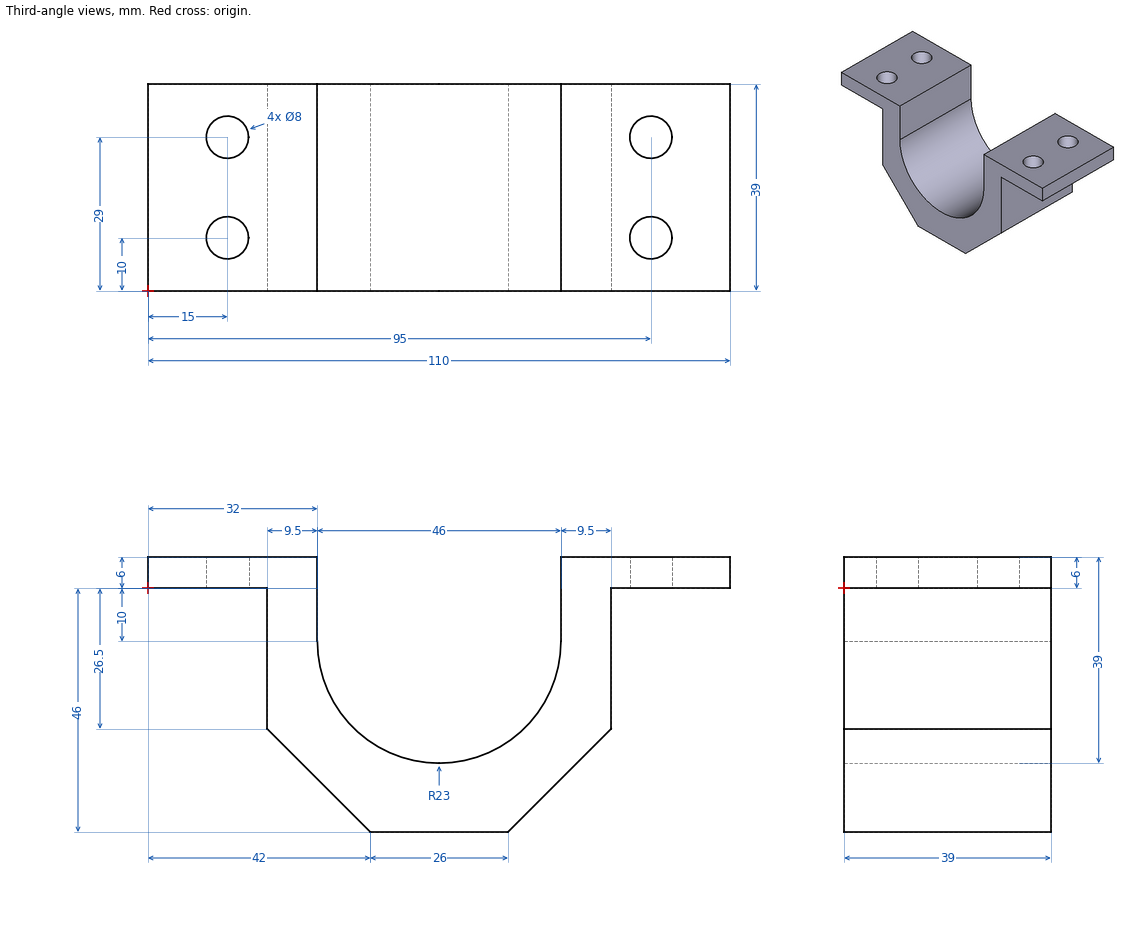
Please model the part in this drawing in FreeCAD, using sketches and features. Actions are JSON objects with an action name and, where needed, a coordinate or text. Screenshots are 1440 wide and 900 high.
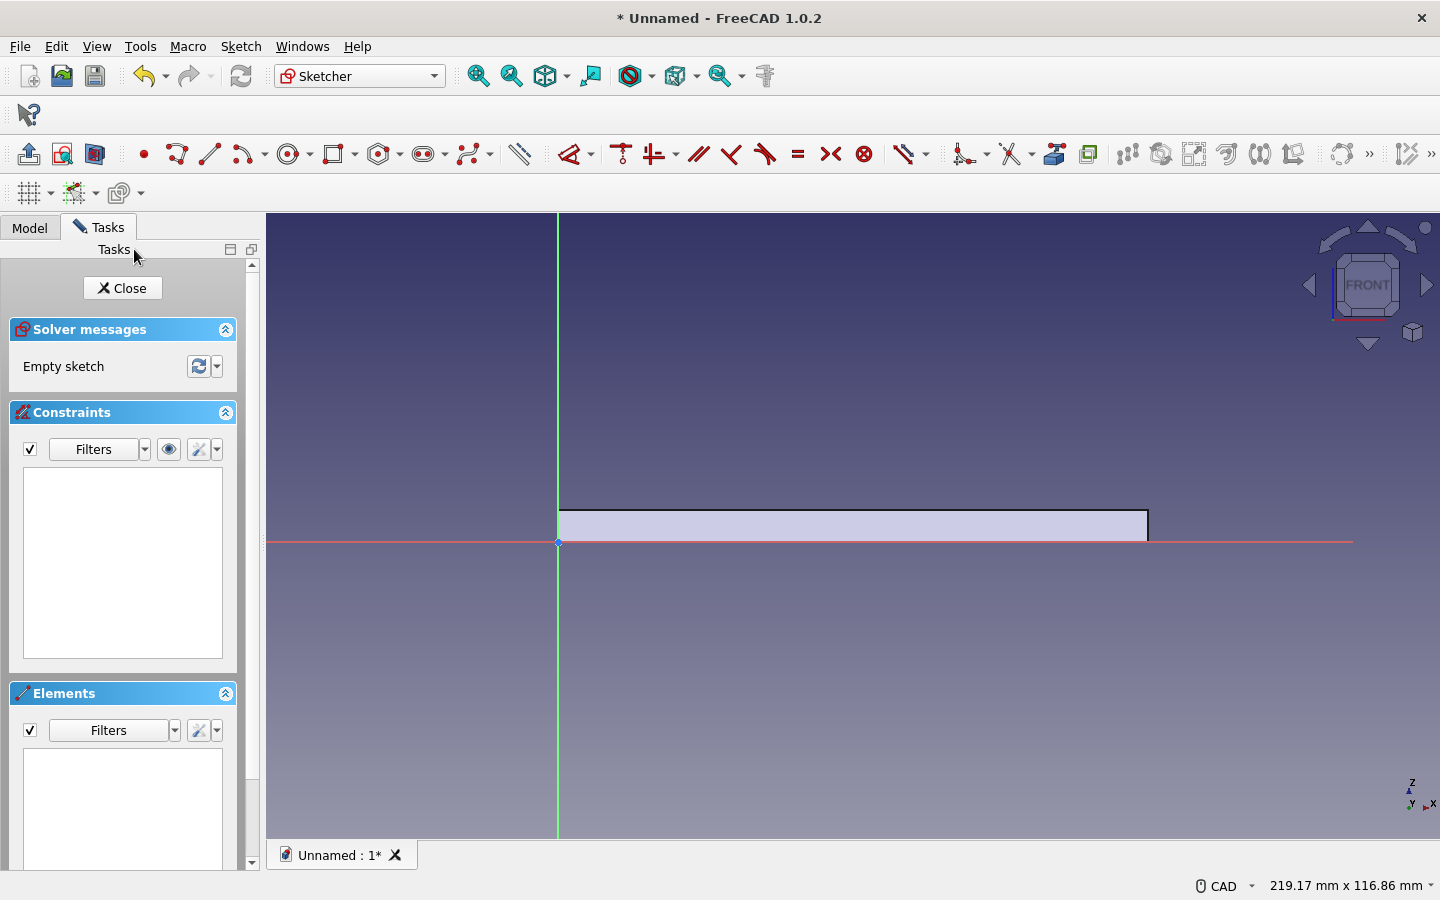
{"action": "scroll", "coordinate": [809, 811], "scroll_direction": "up", "scroll_amount": 2}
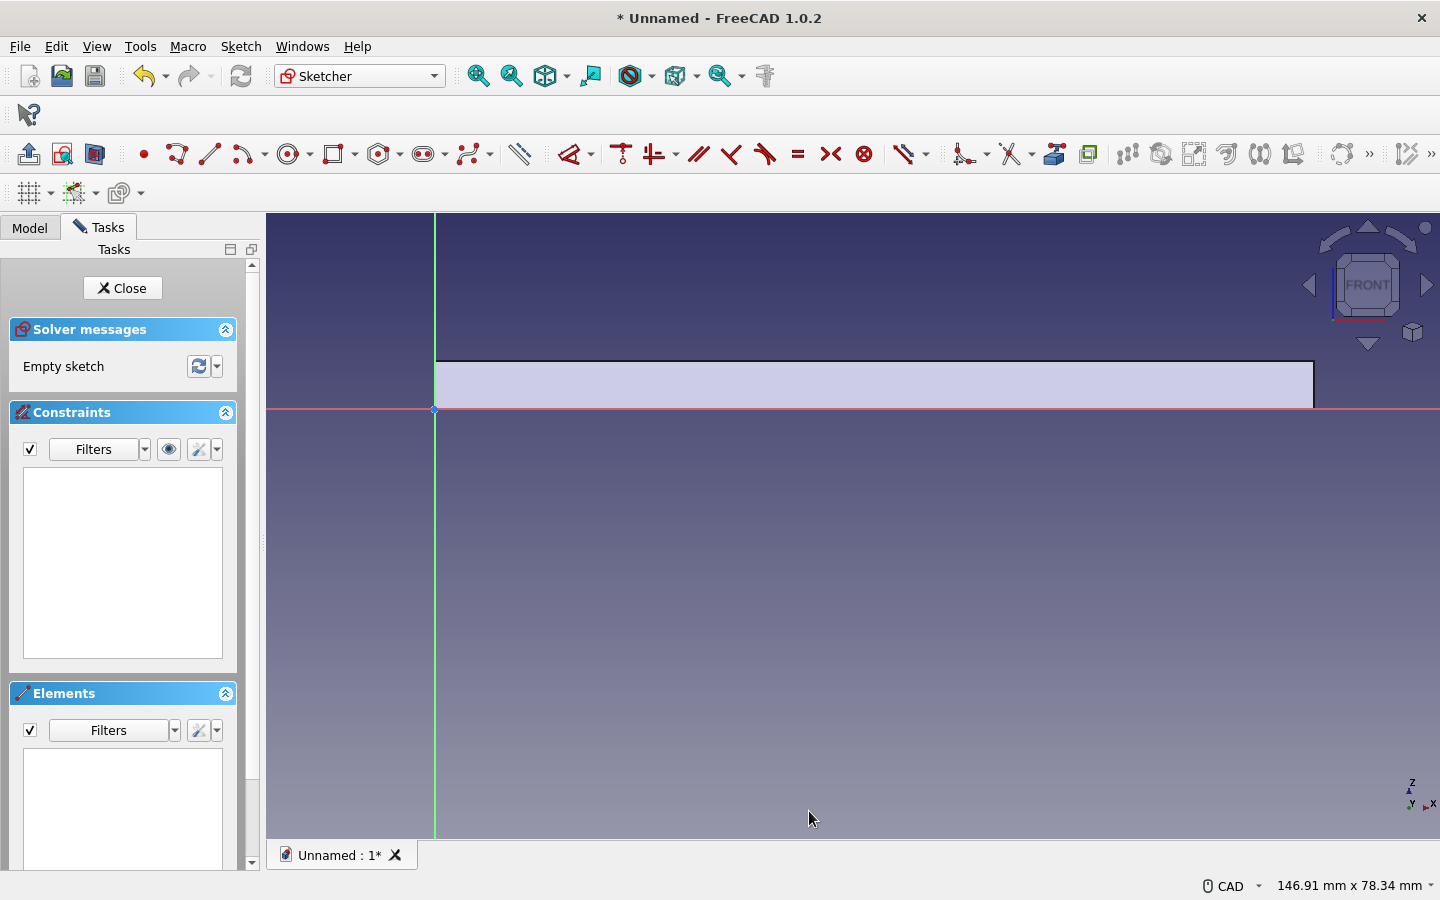
{"action": "left_click", "coordinate": [177, 154]}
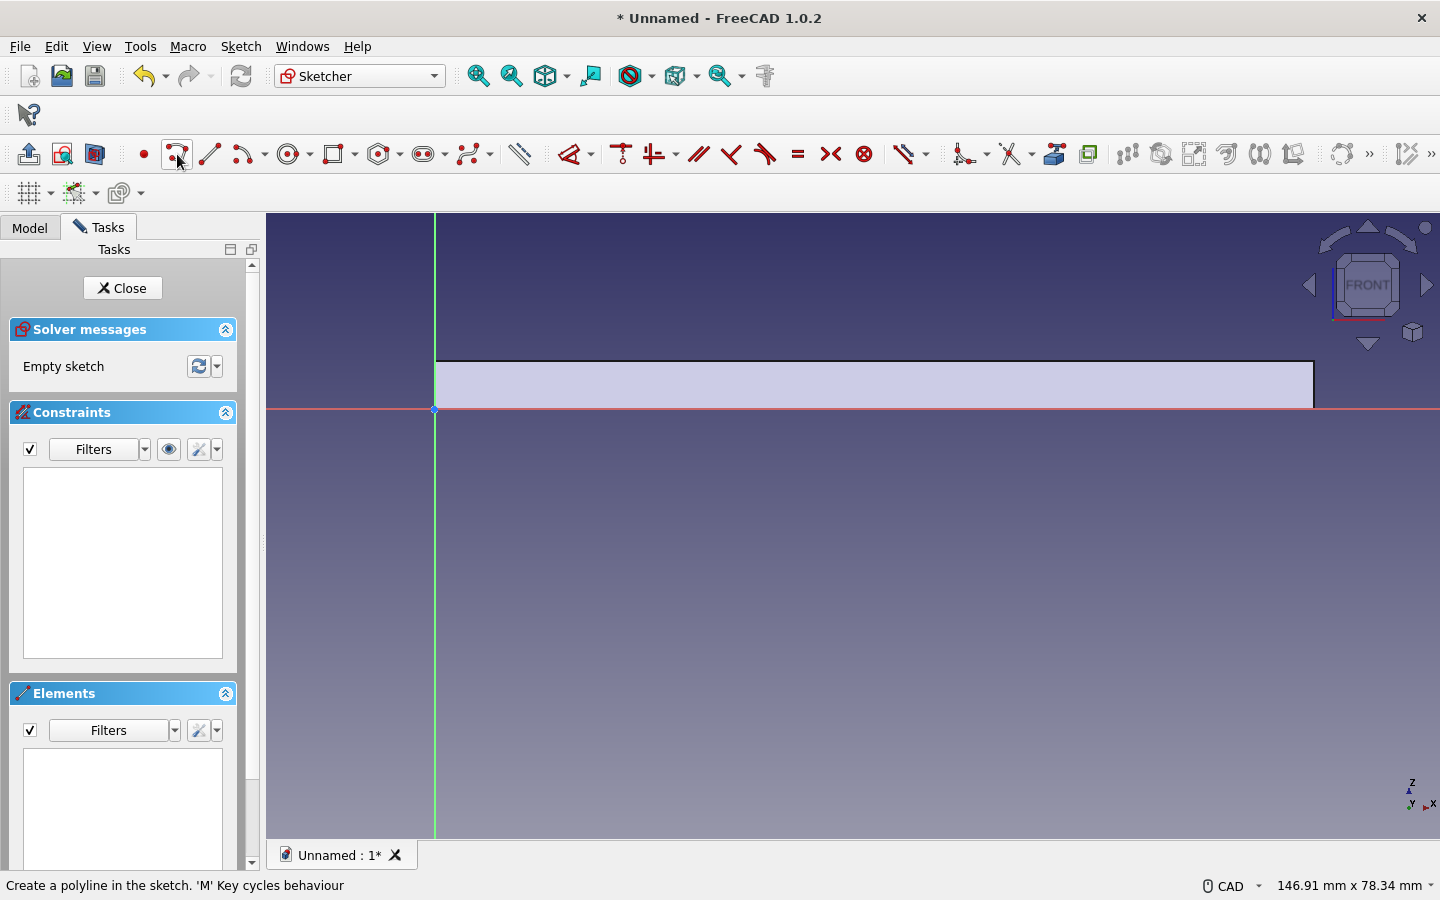
{"action": "left_click", "coordinate": [691, 489]}
{"action": "left_click", "coordinate": [691, 409]}
{"action": "left_click", "coordinate": [615, 418]}
{"action": "left_click", "coordinate": [615, 621]}
{"action": "left_click", "coordinate": [771, 777]}
{"action": "left_click", "coordinate": [978, 777]}
{"action": "left_click", "coordinate": [1134, 621]}
{"action": "left_click", "coordinate": [1134, 409]}
{"action": "left_click", "coordinate": [1058, 418]}
{"action": "left_click", "coordinate": [1058, 489]}
{"action": "right_click", "coordinate": [1058, 489]}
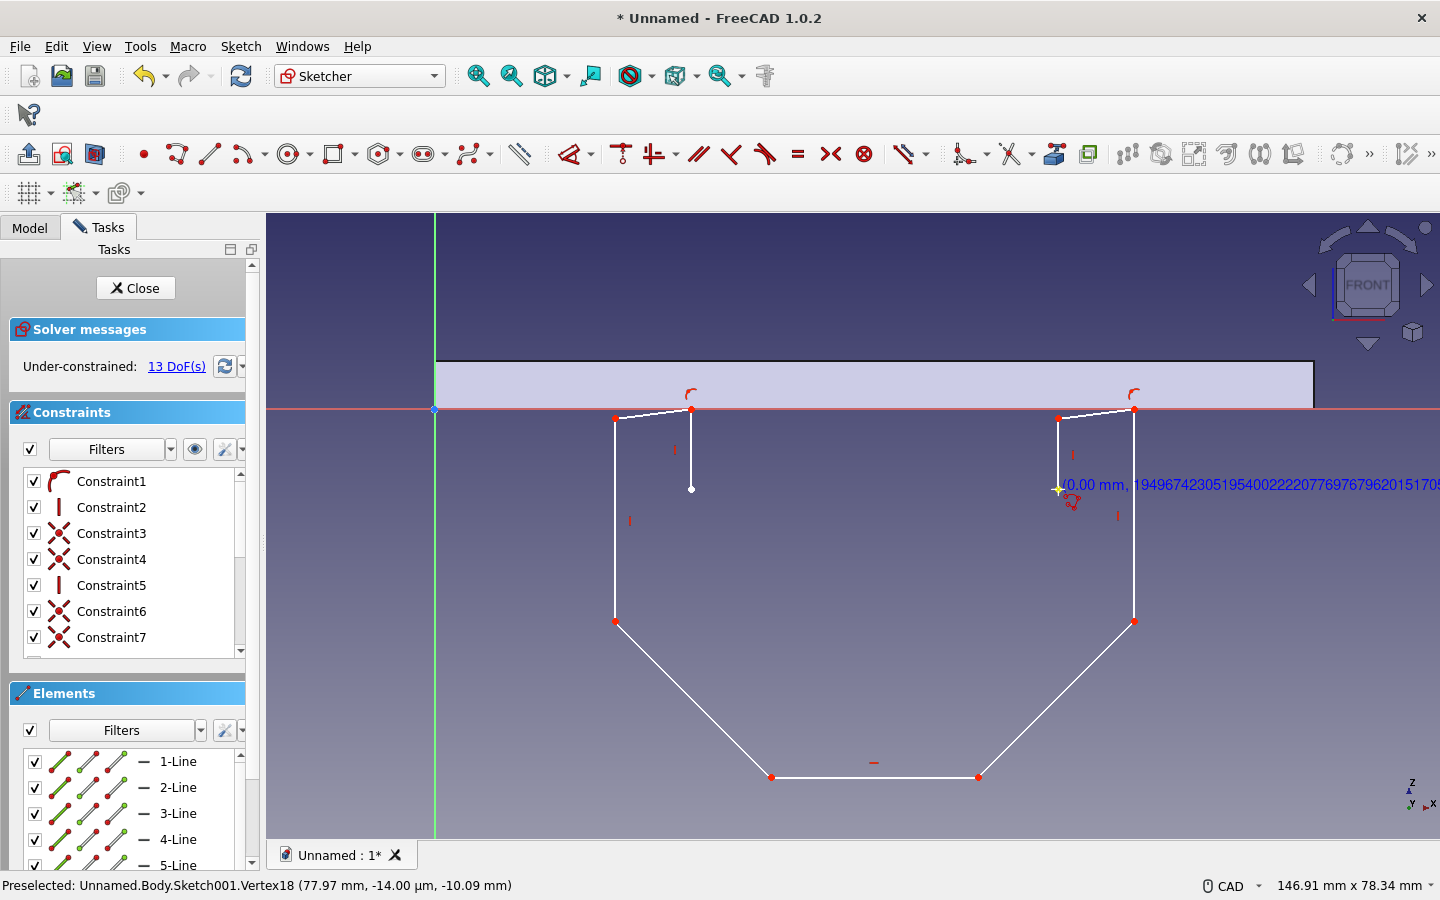
{"action": "key", "text": "g 3 a"}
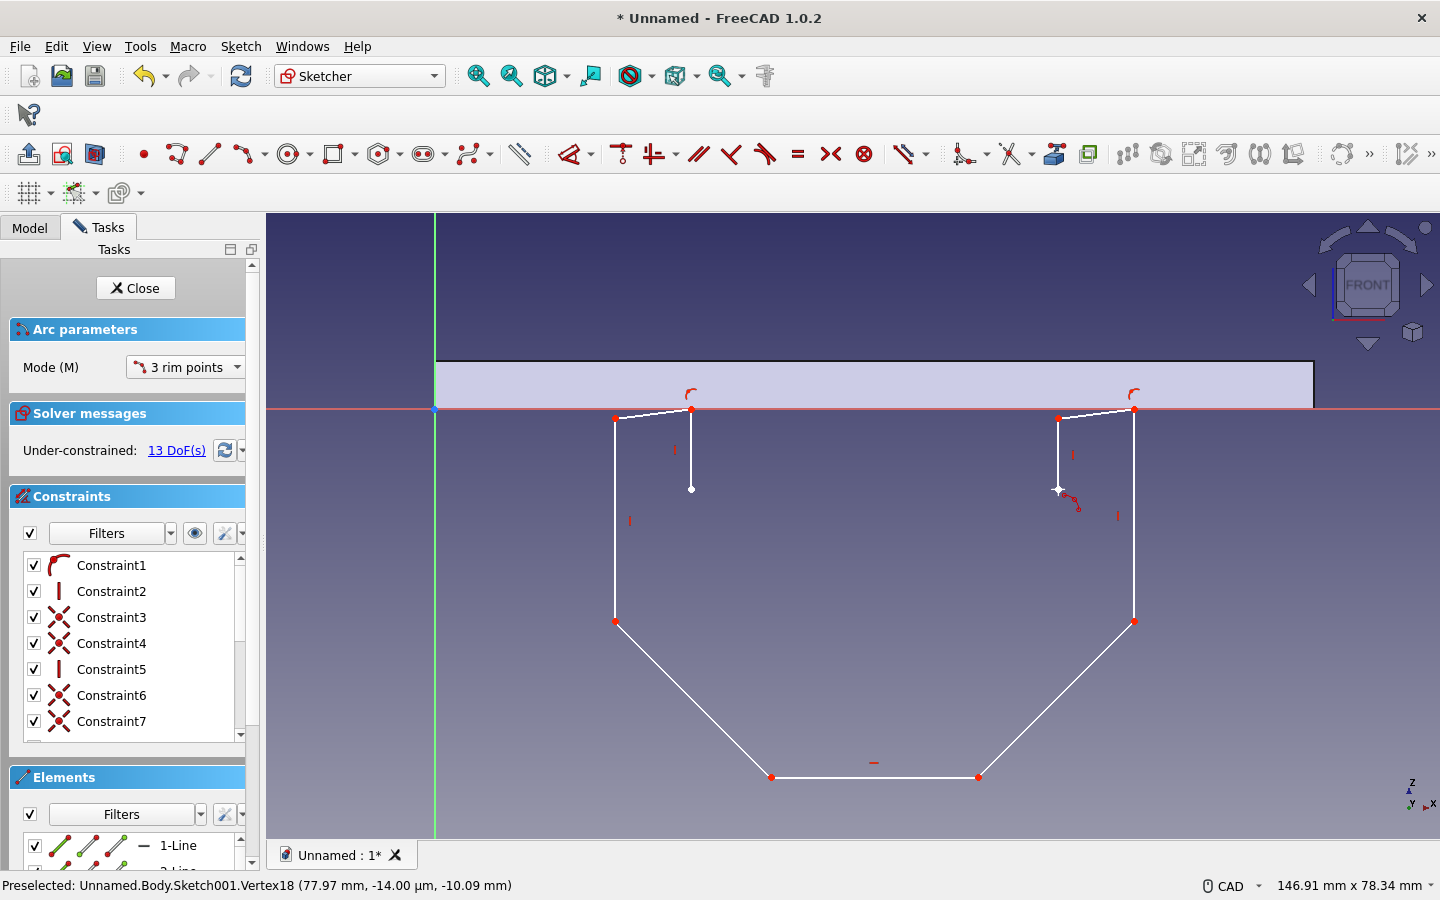
{"action": "left_click", "coordinate": [1058, 490]}
{"action": "left_click", "coordinate": [691, 490]}
{"action": "left_click", "coordinate": [874, 673]}
{"action": "key", "text": "Escape"}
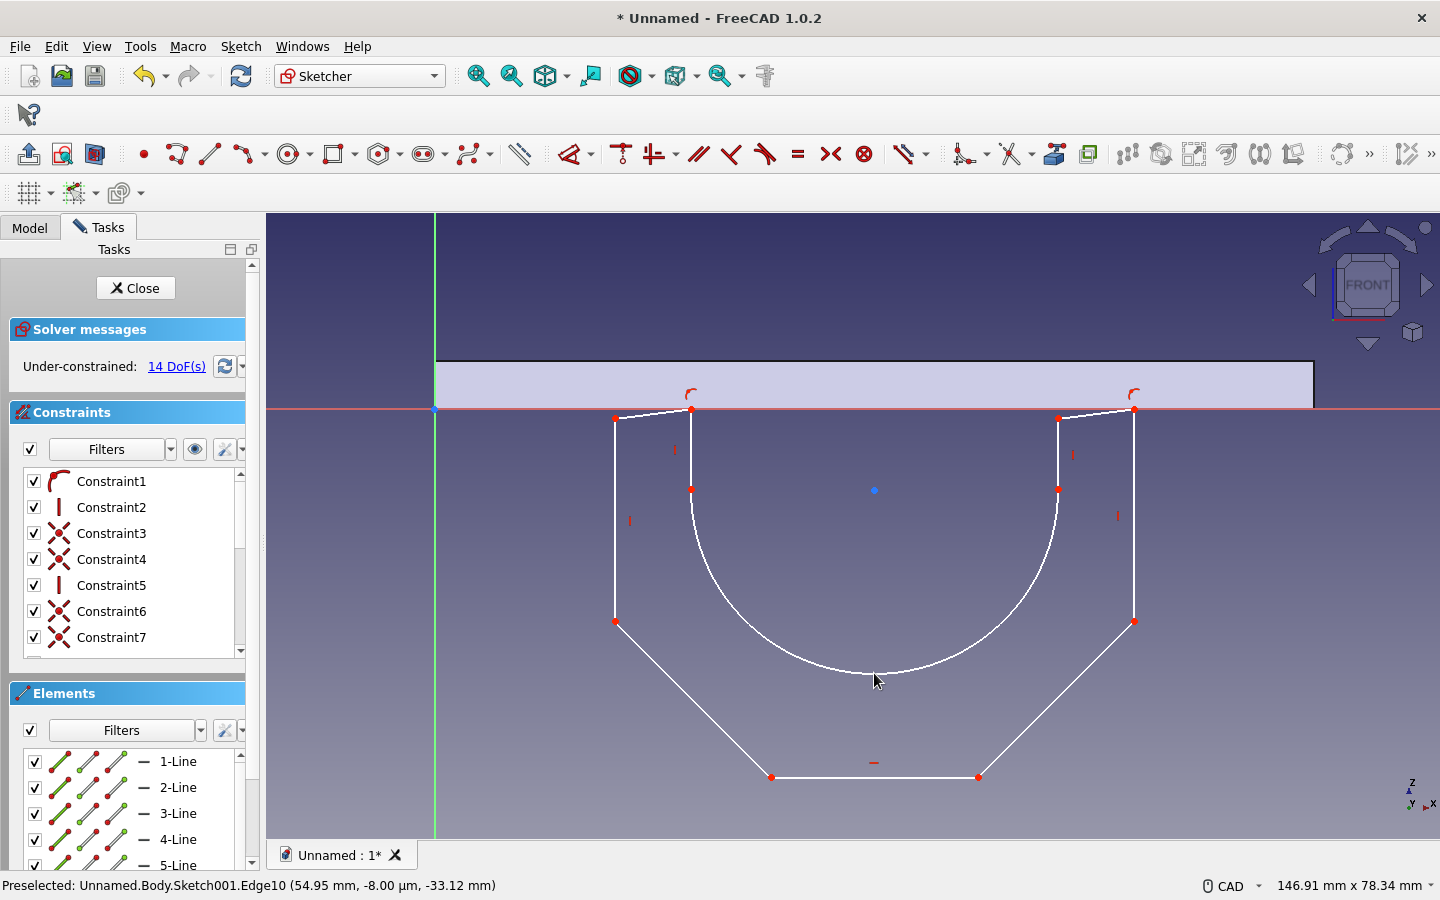
{"action": "left_click", "coordinate": [691, 466]}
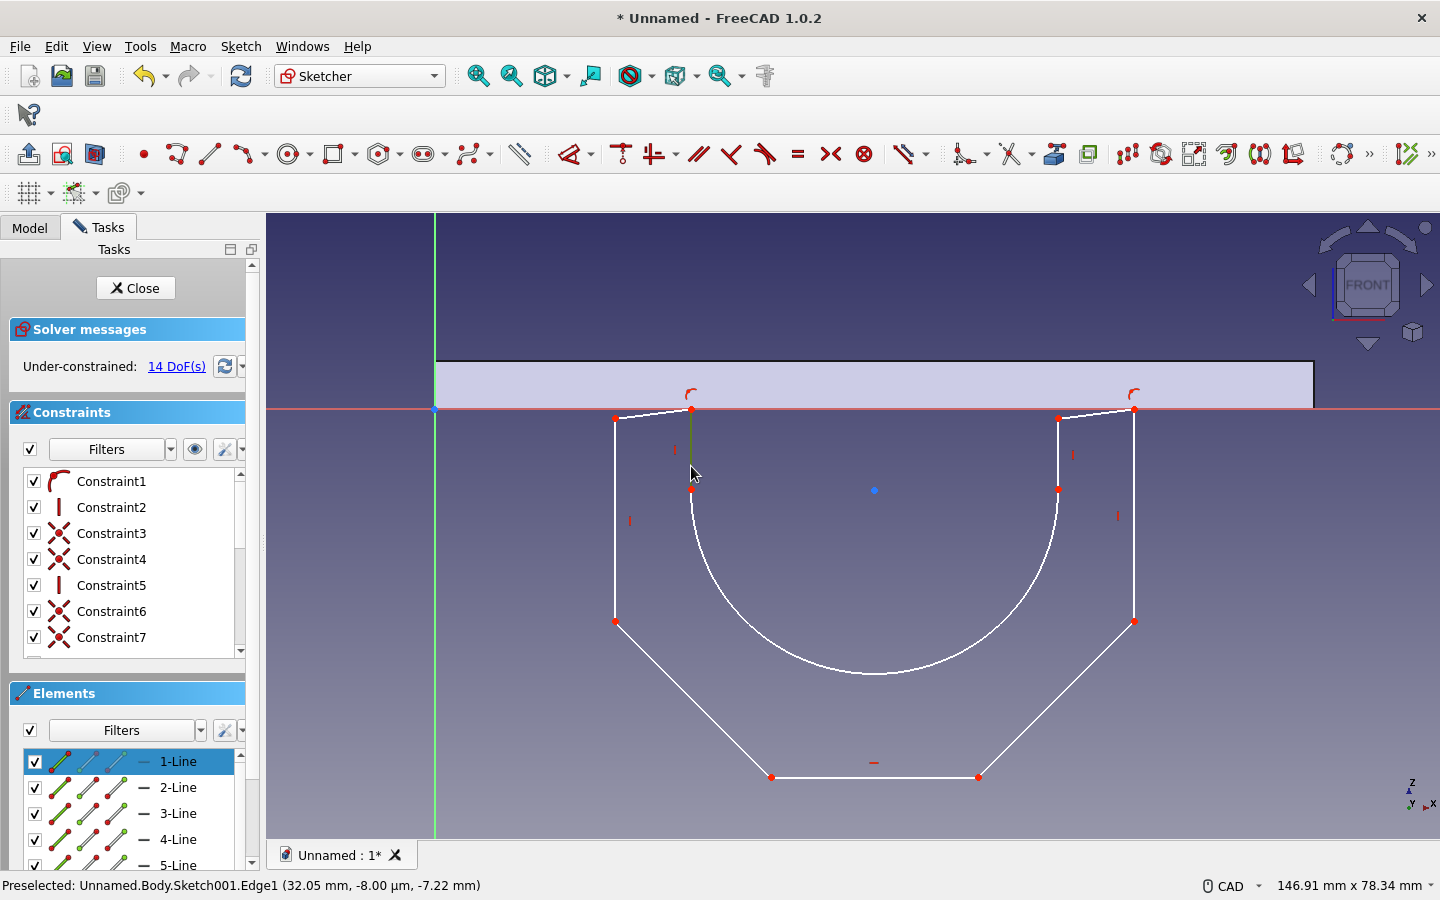
{"action": "left_click", "coordinate": [766, 639]}